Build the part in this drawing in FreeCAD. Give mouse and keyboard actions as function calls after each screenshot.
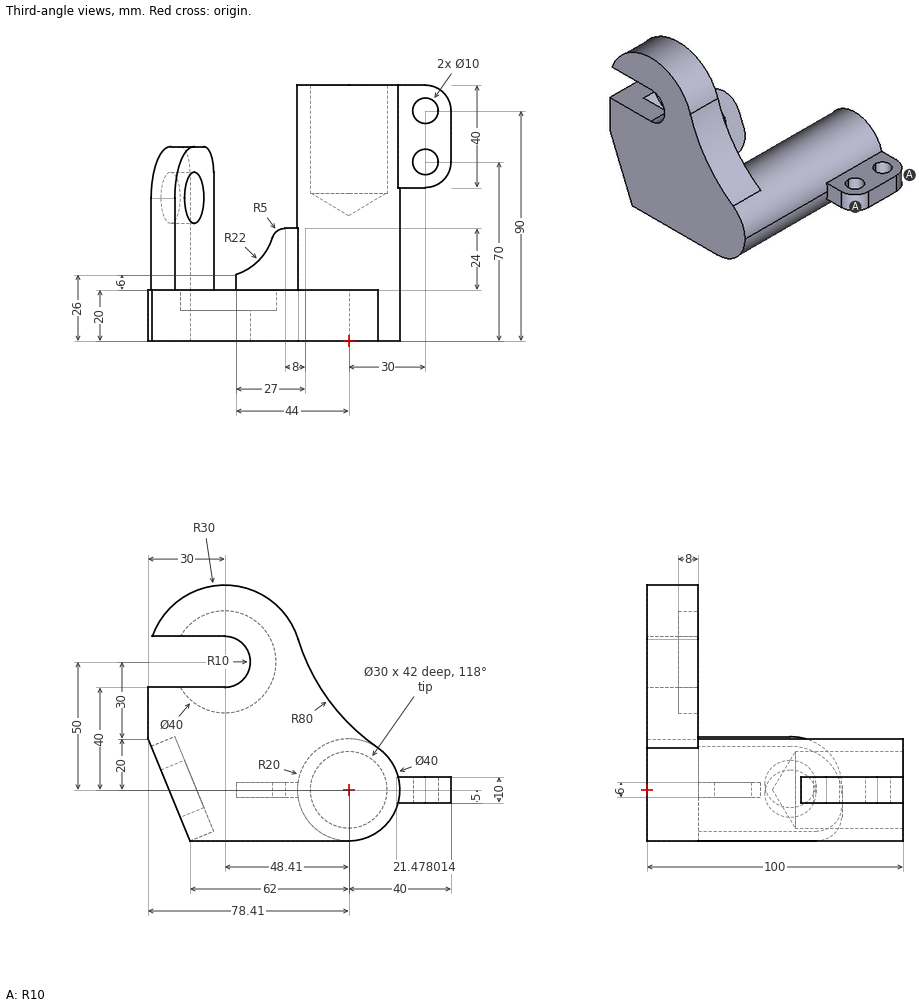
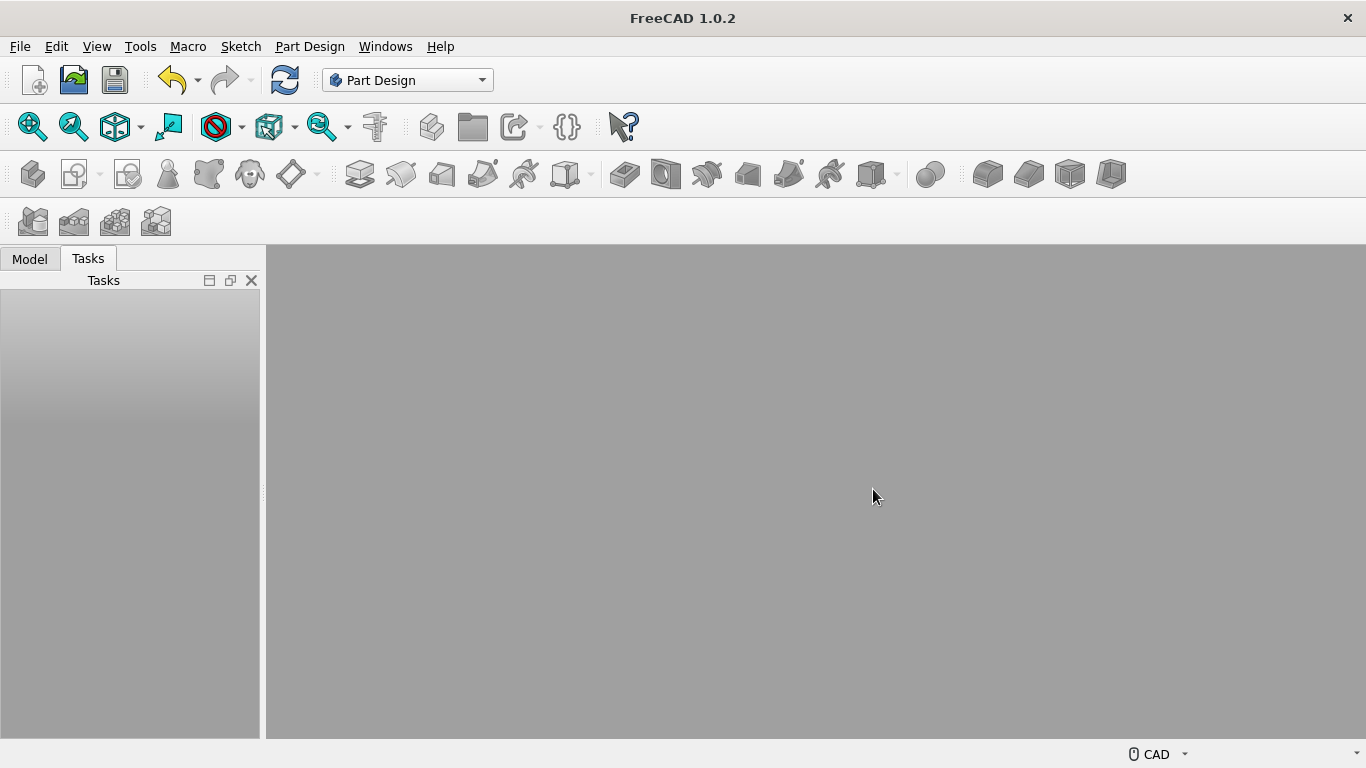
click(33, 80)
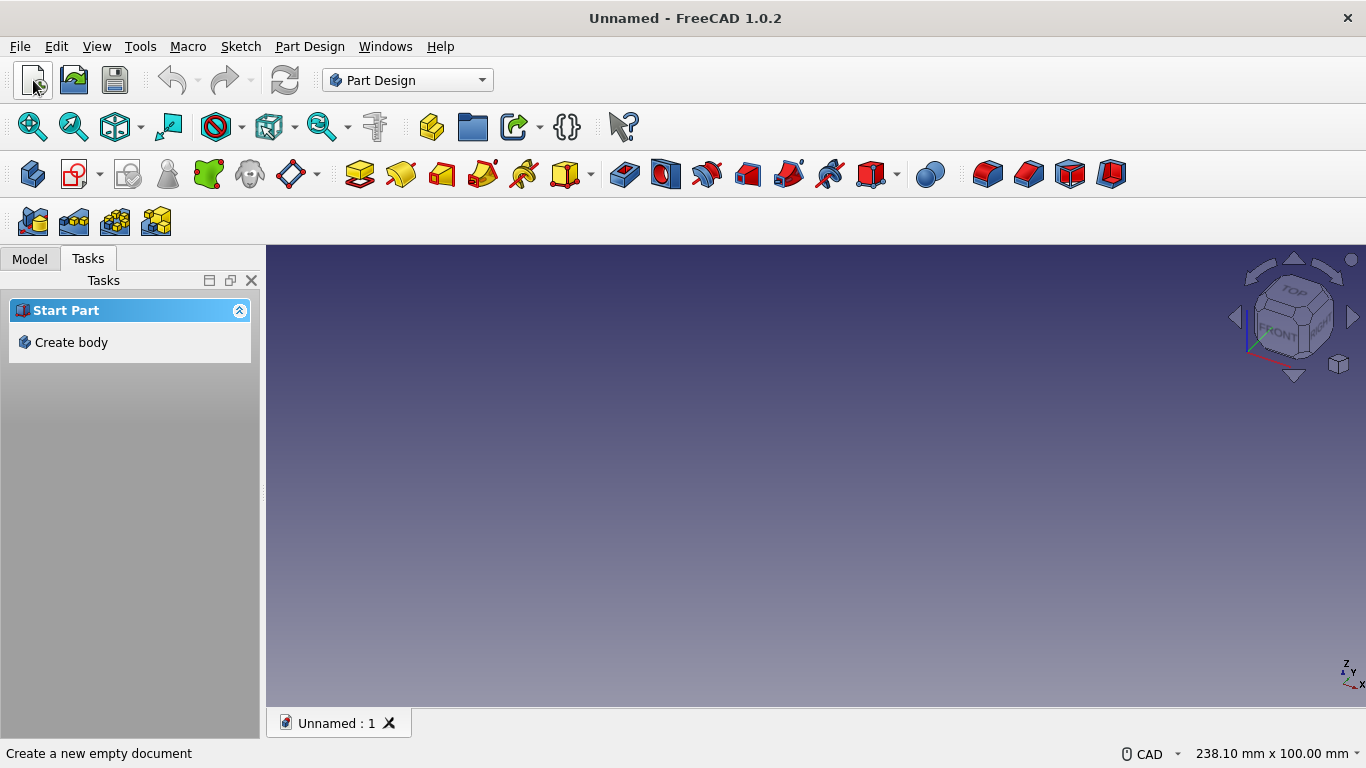
click(74, 174)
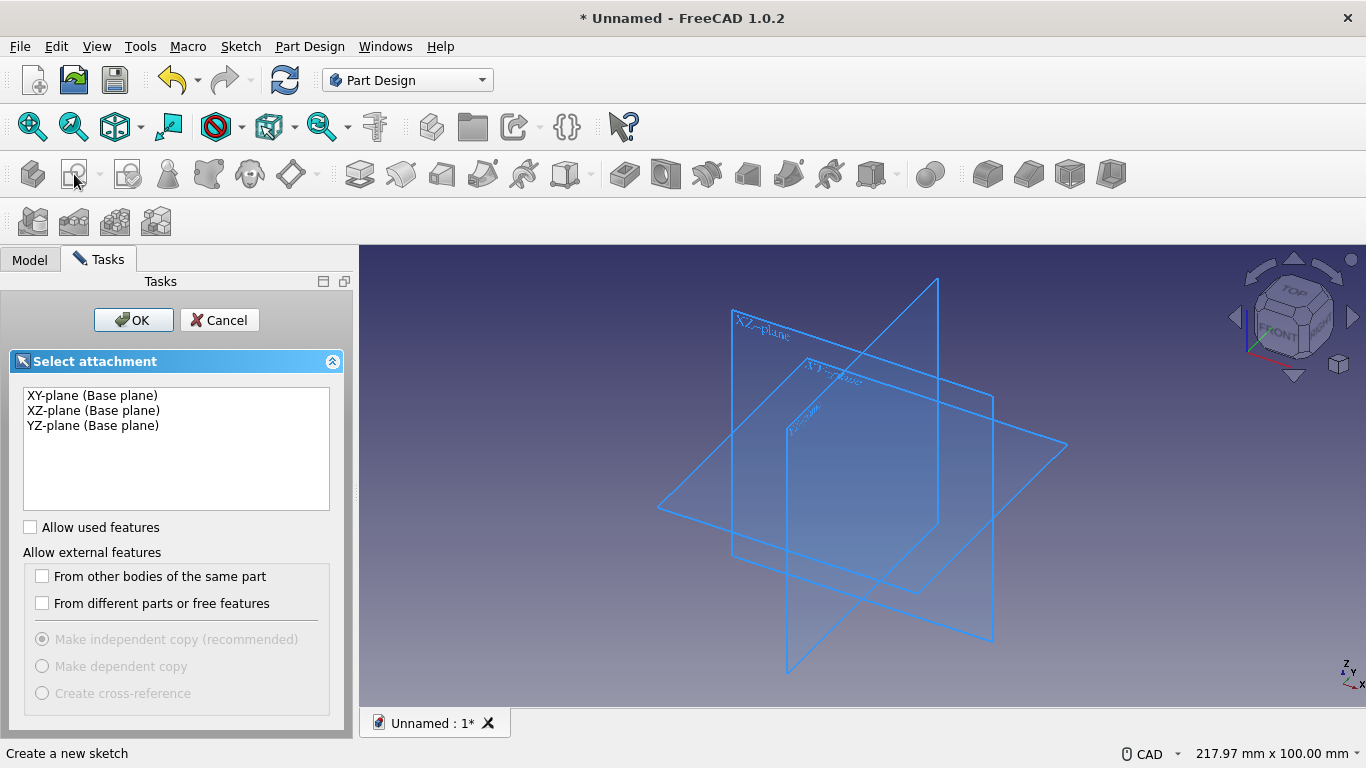
click(84, 410)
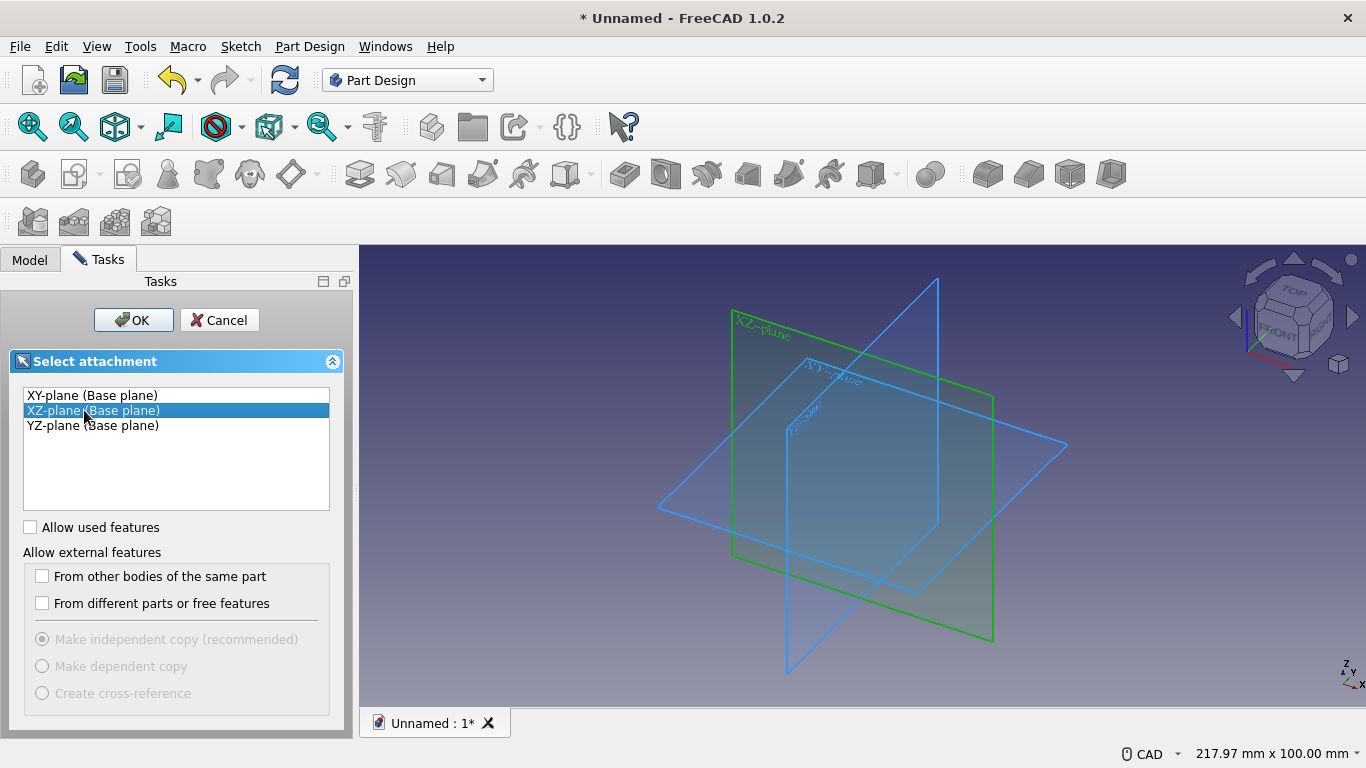
click(134, 320)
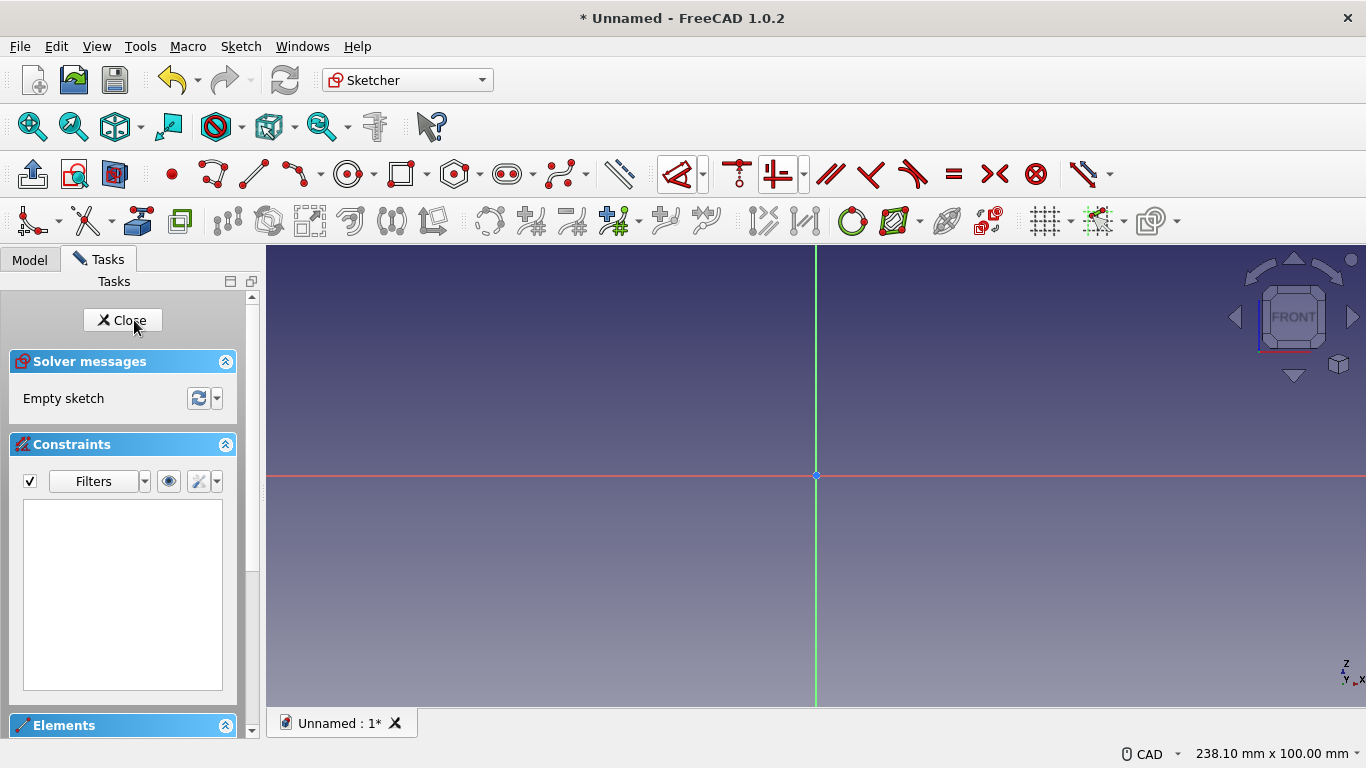
scroll(955, 476, up, 2)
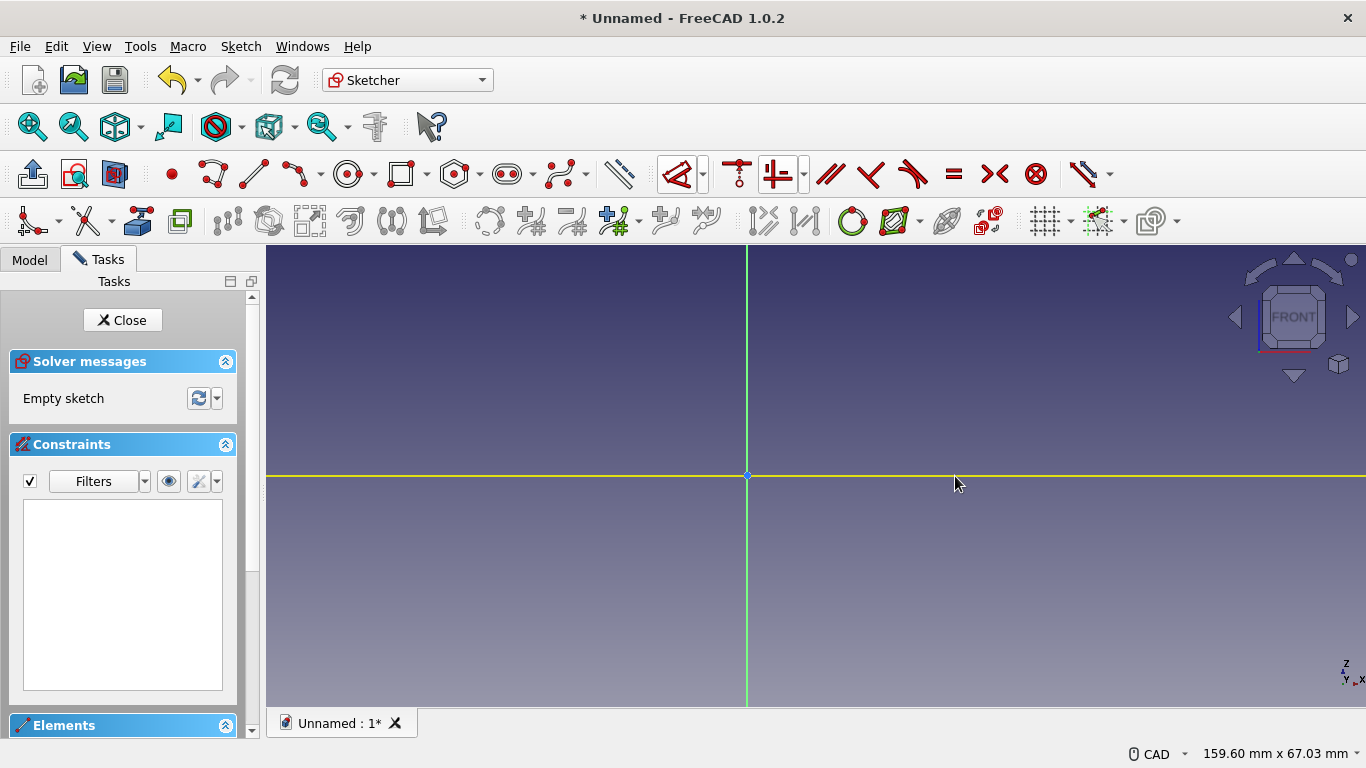
key(g)
key(c)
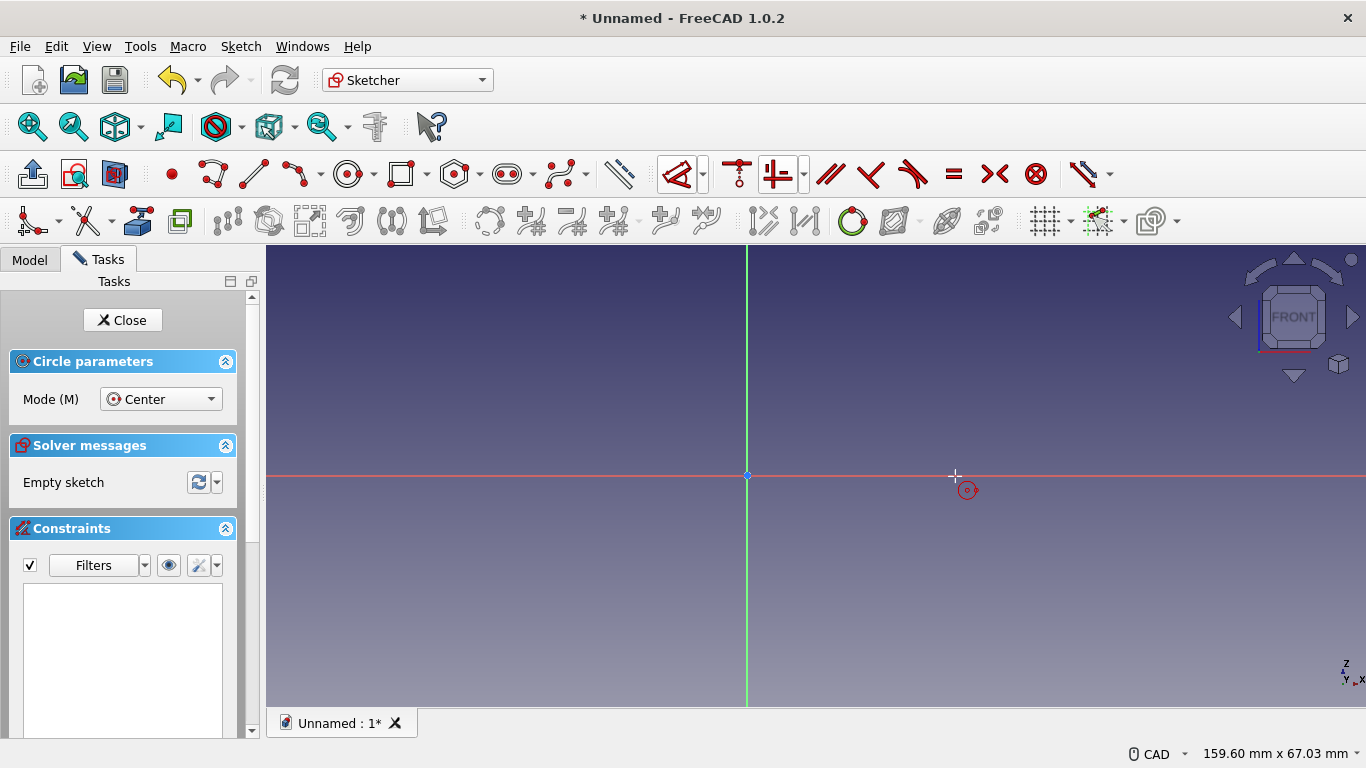
click(747, 476)
click(845, 378)
key(Escape)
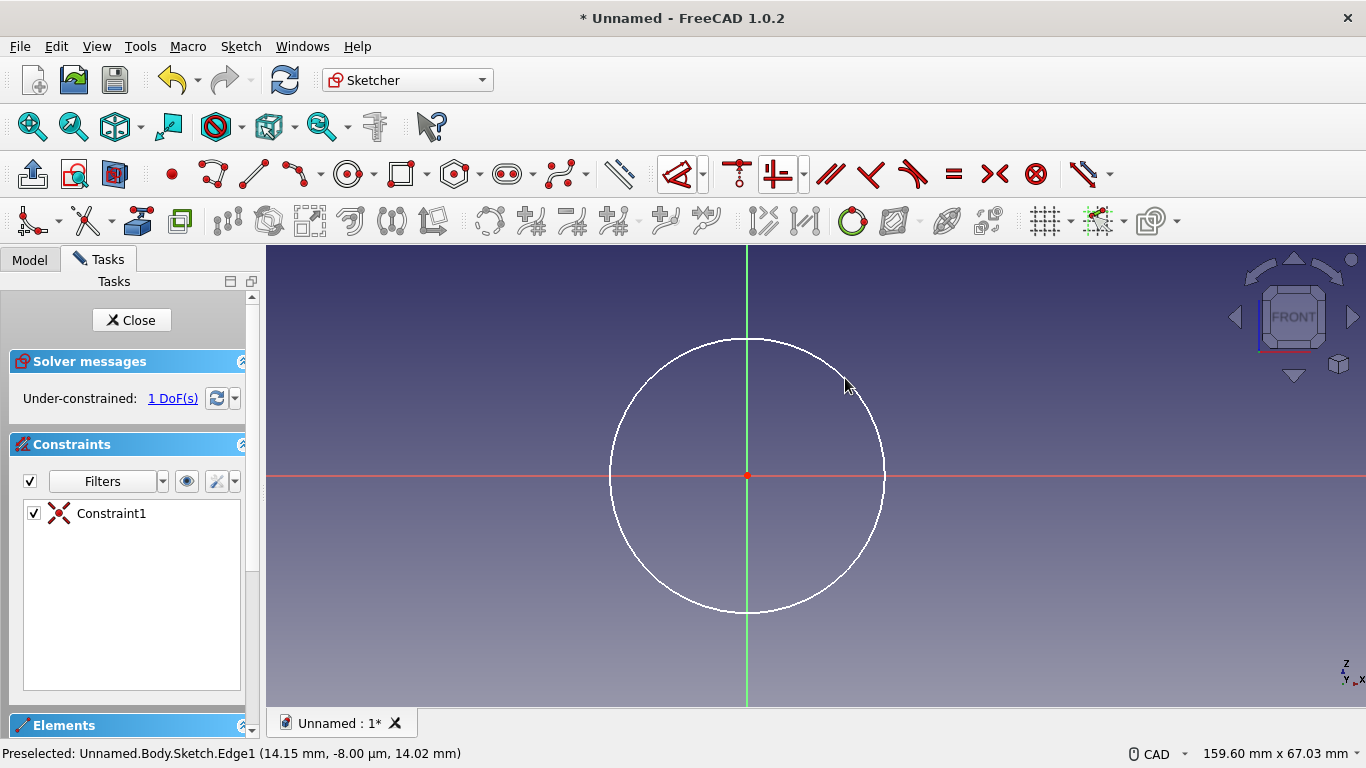
key(d)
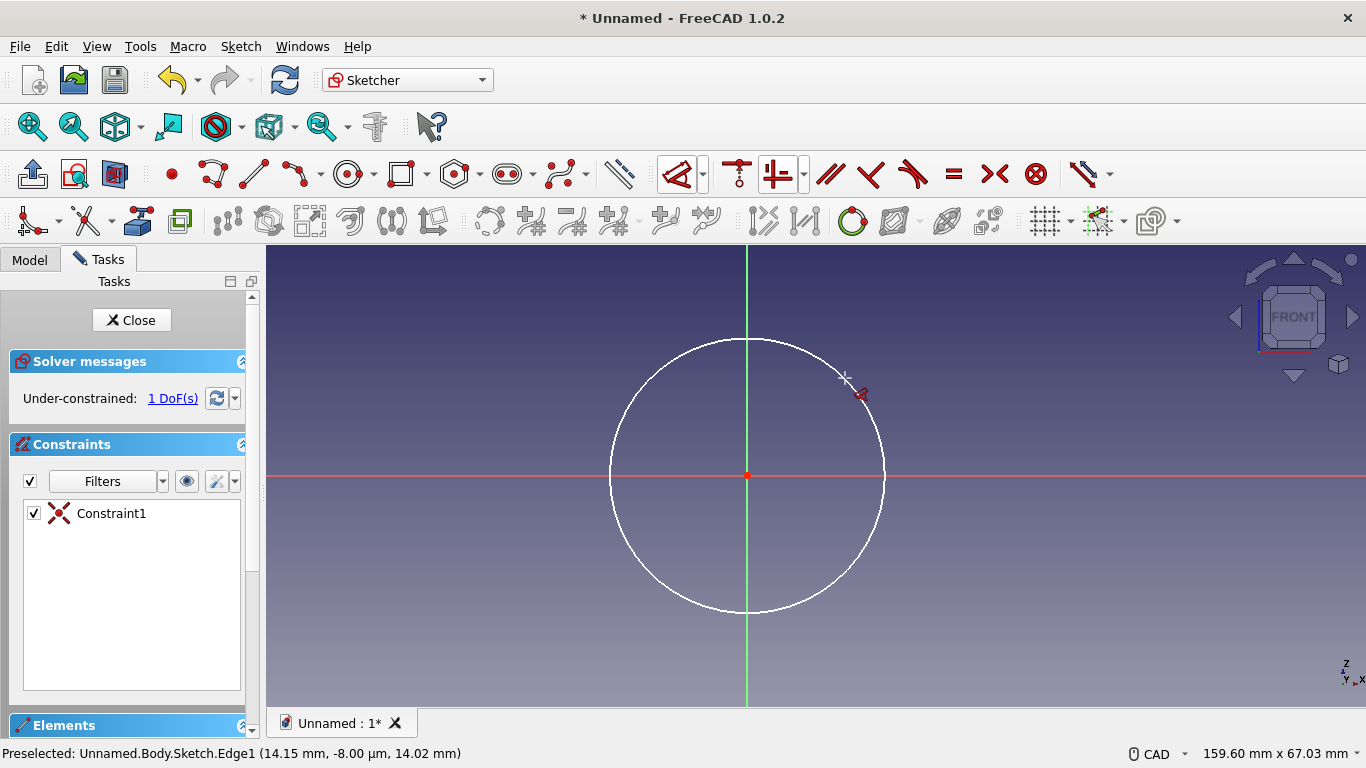
click(844, 378)
click(867, 355)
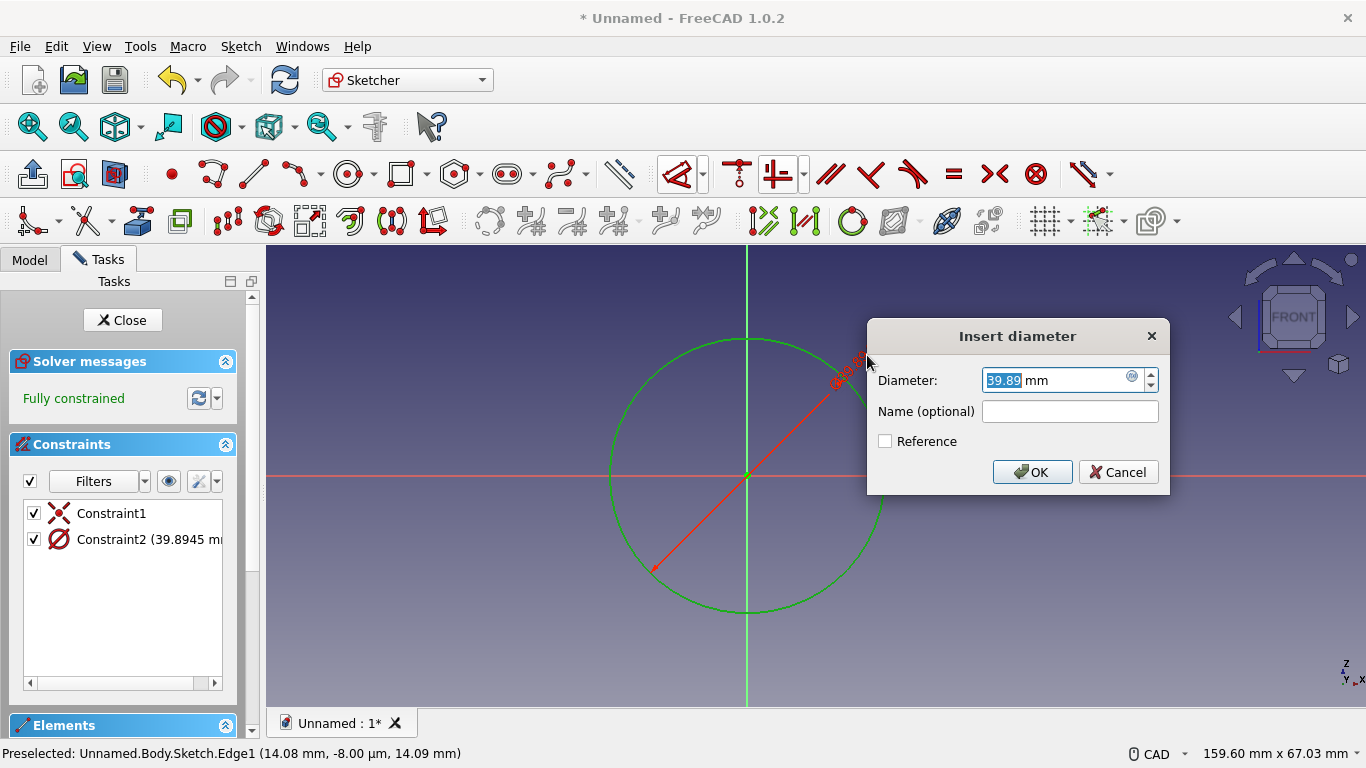
text(40)
key(Return)
key(Escape)